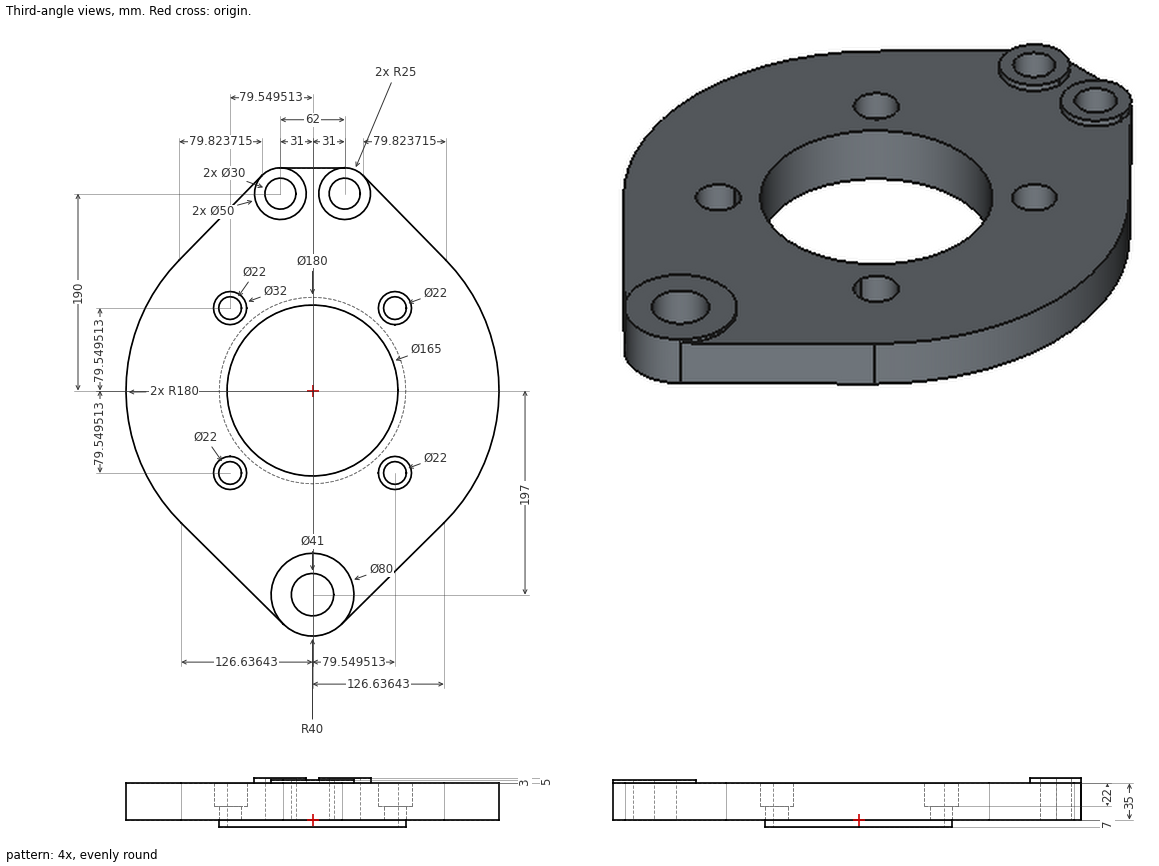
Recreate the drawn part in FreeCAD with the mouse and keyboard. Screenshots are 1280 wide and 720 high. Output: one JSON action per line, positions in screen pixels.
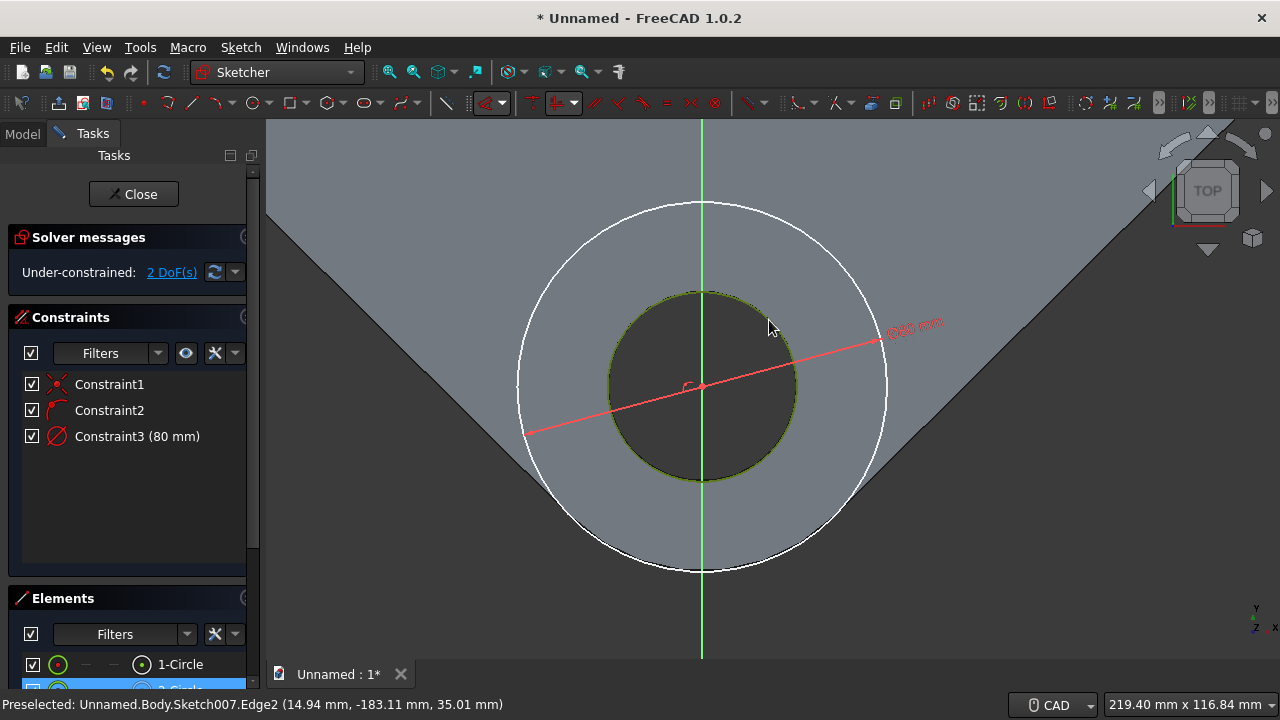
{"action": "key", "text": "k o"}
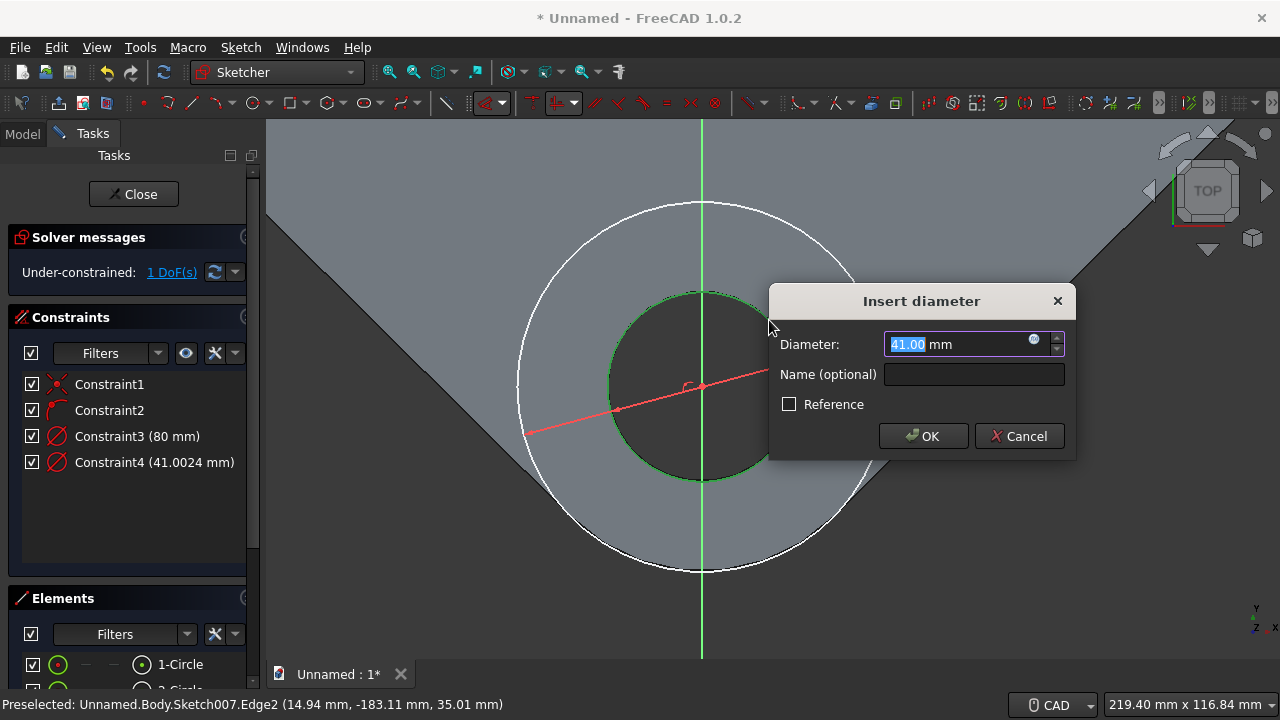
{"action": "type", "text": "41"}
{"action": "key", "text": "Return"}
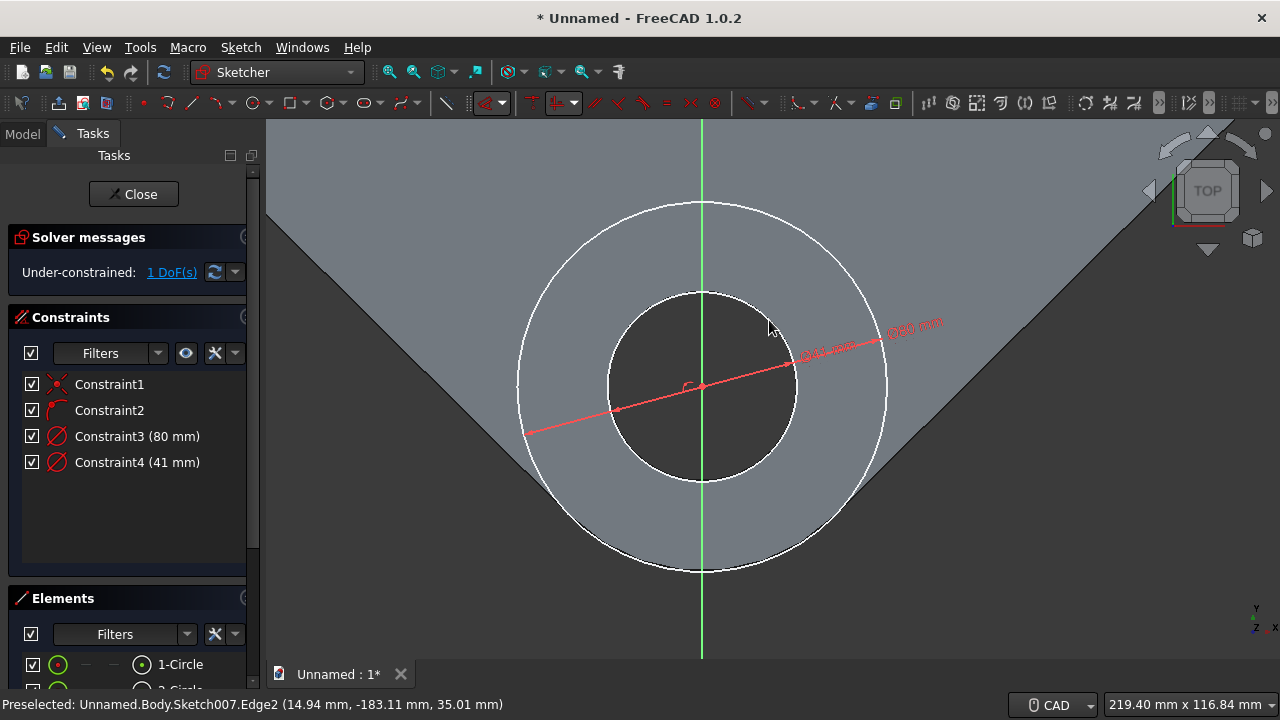
{"action": "left_click", "coordinate": [702, 387]}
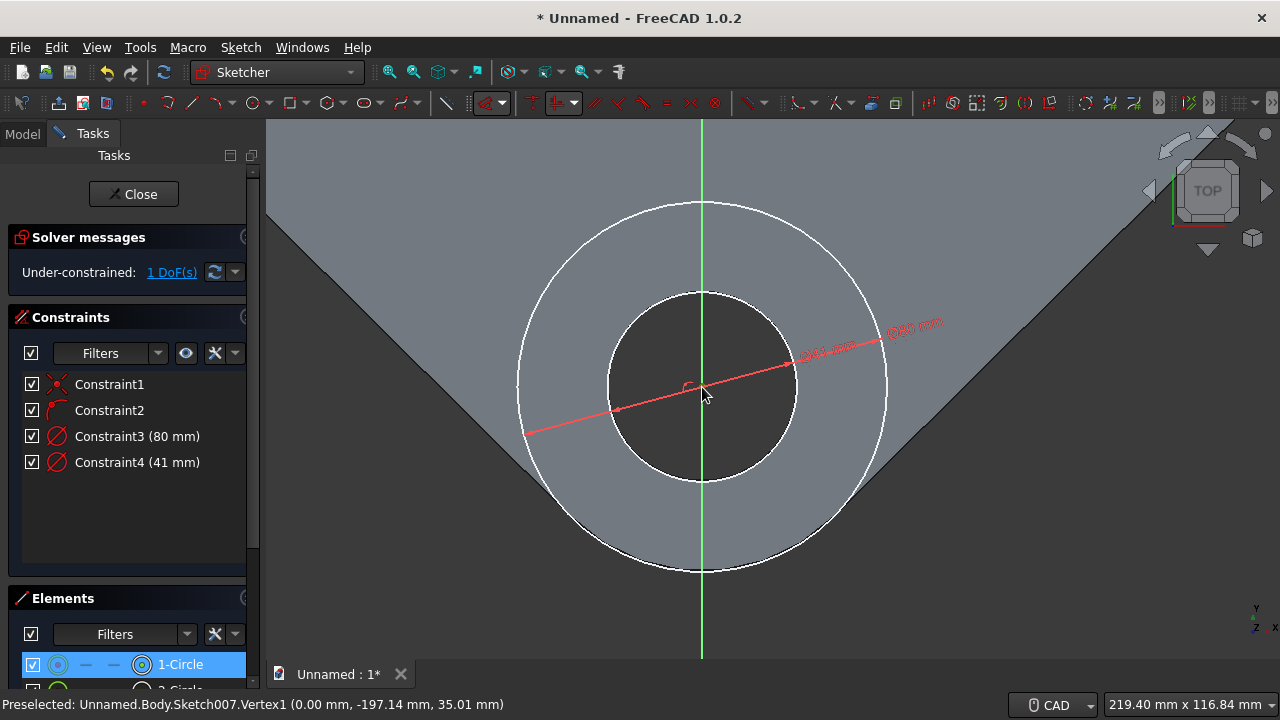
{"action": "key", "text": "i"}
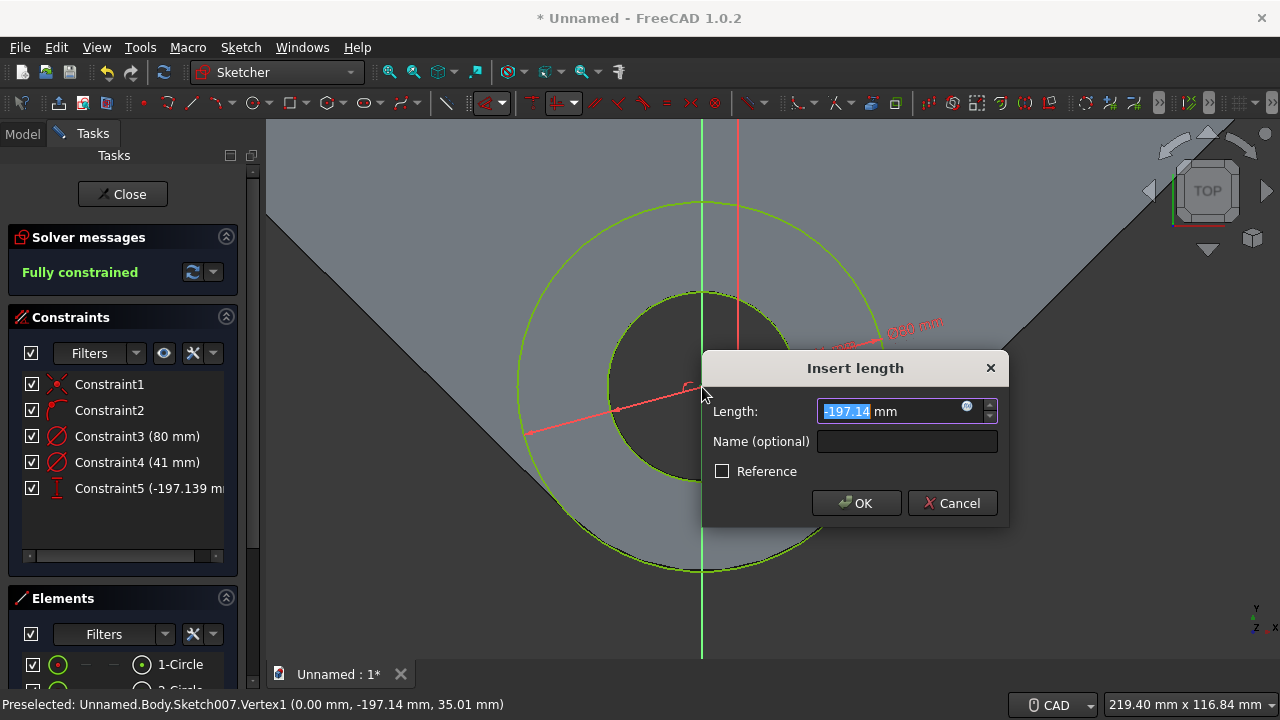
{"action": "type", "text": "-197"}
{"action": "key", "text": "Return"}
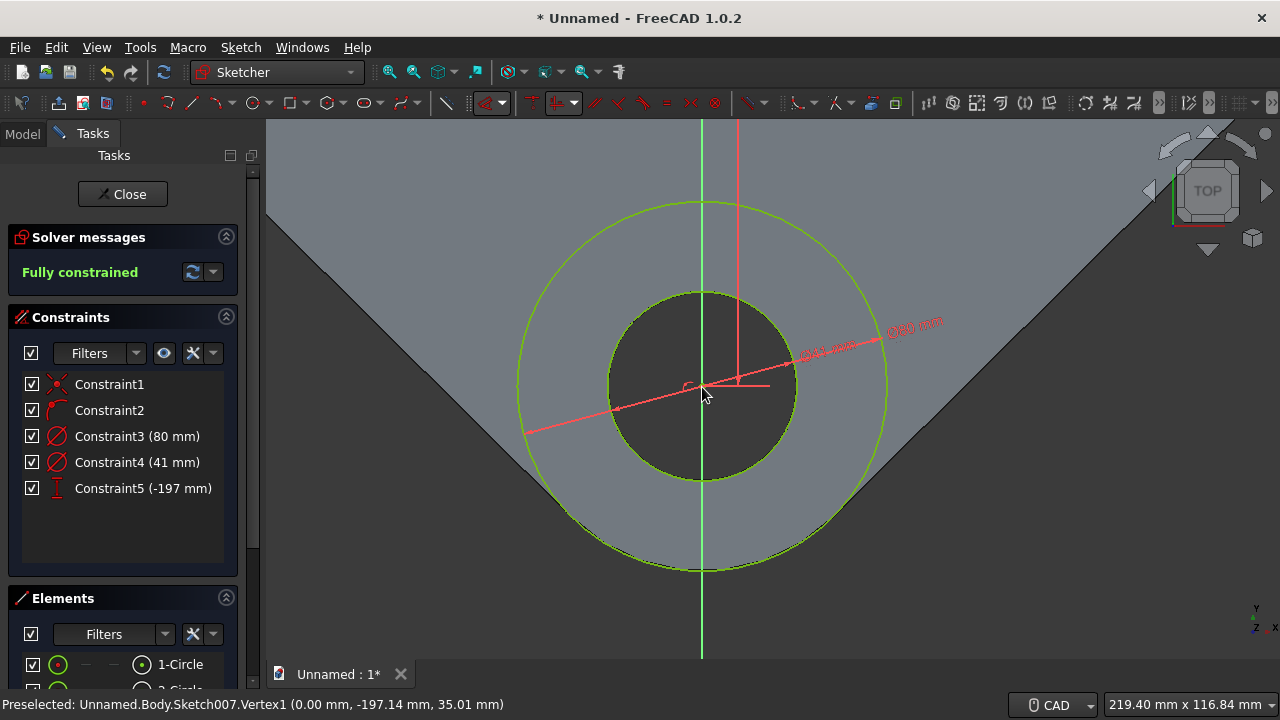
{"action": "left_click", "coordinate": [123, 194]}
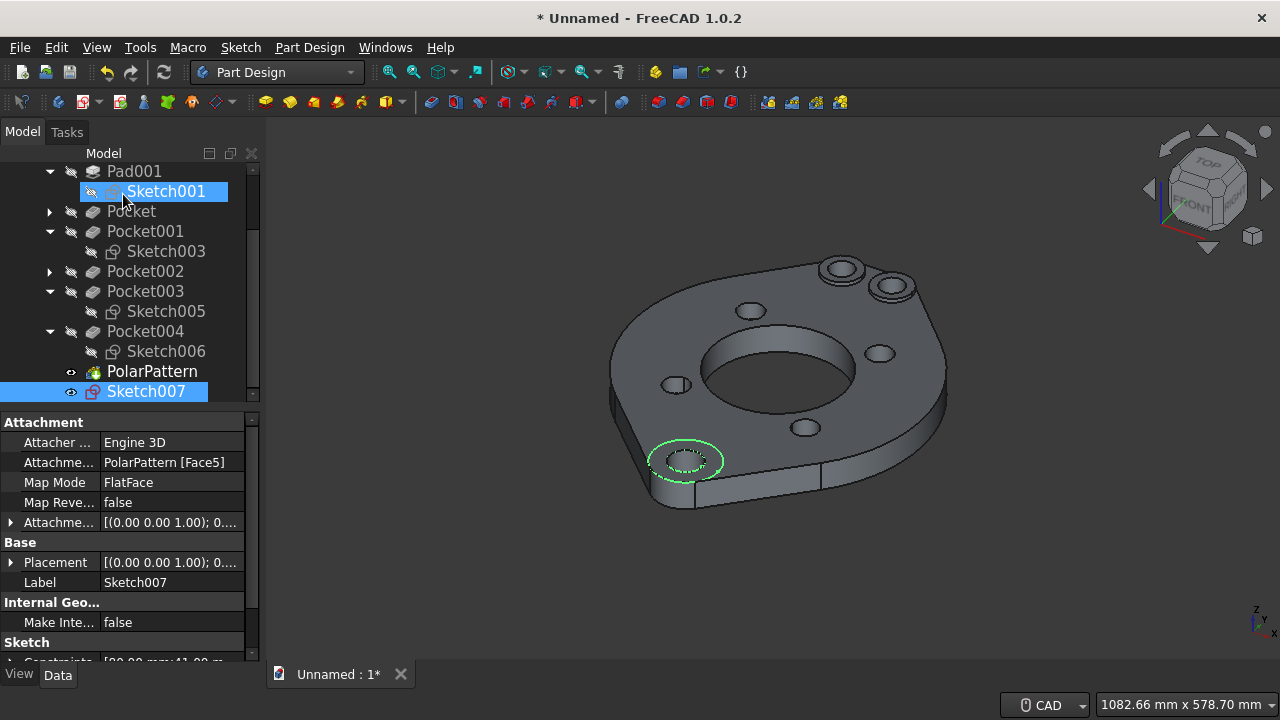
{"action": "left_click", "coordinate": [266, 102]}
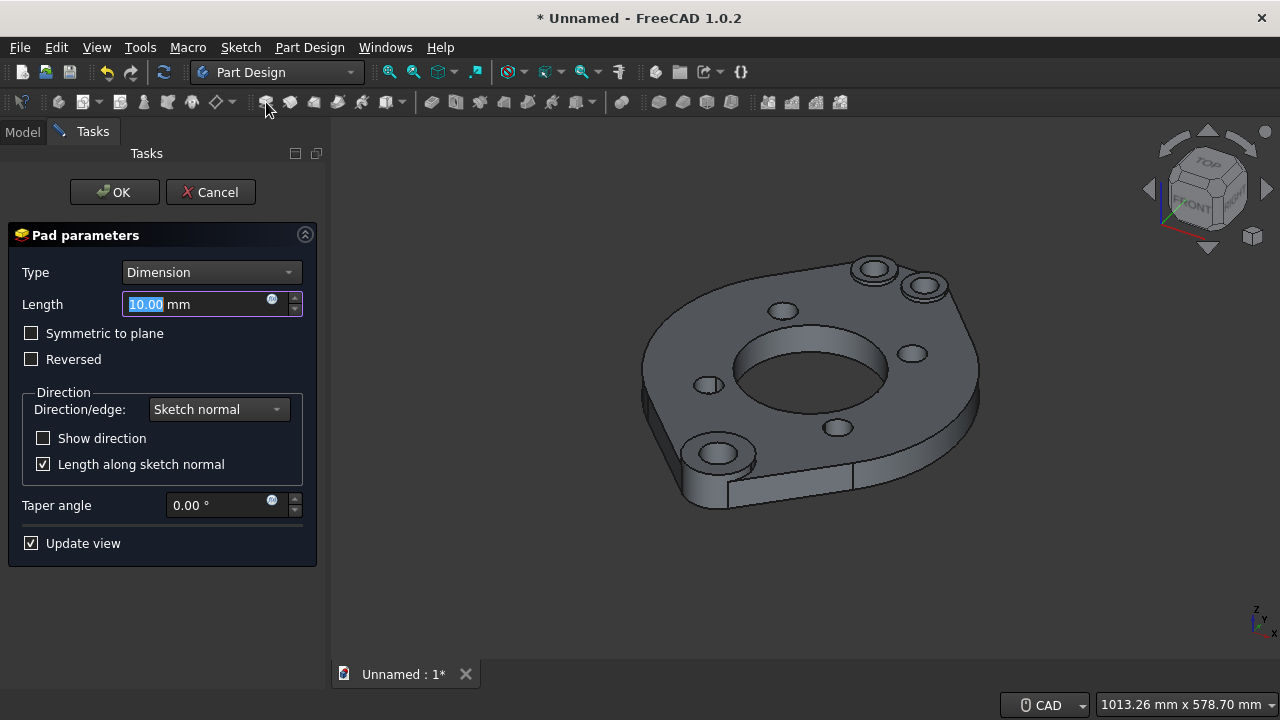
{"action": "type", "text": "3"}
{"action": "key", "text": "Tab"}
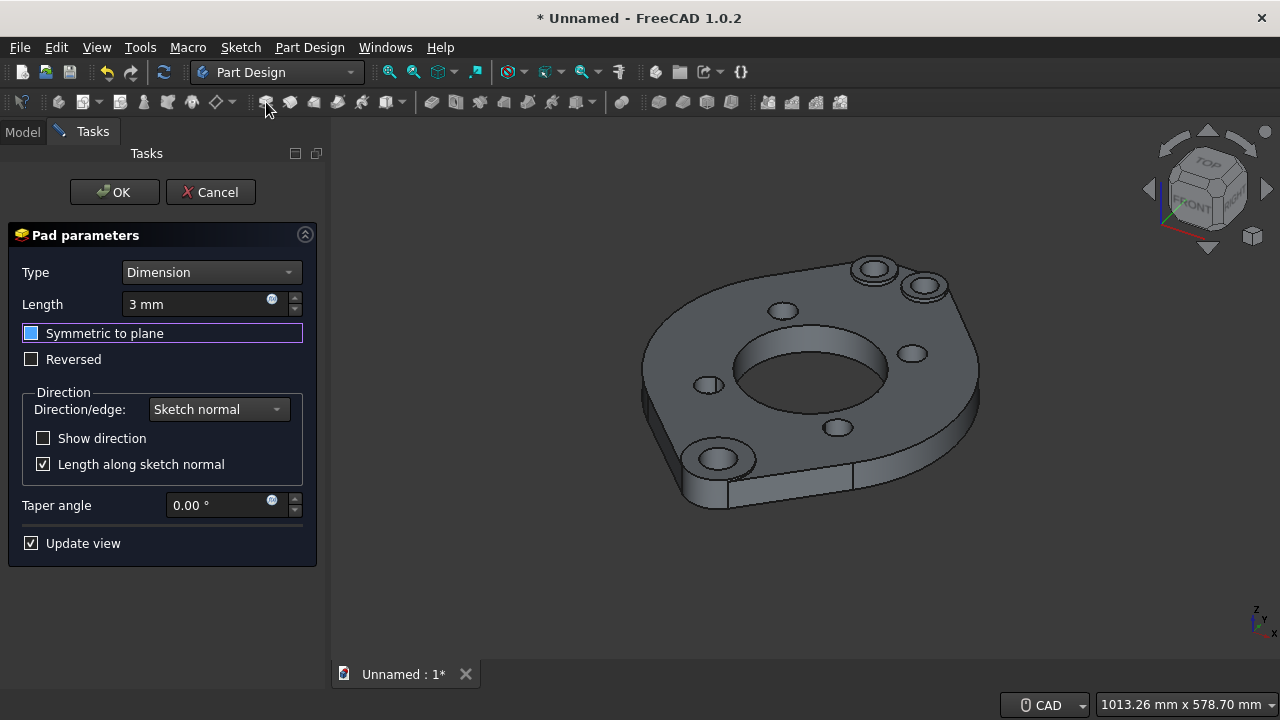
{"action": "left_click", "coordinate": [115, 192]}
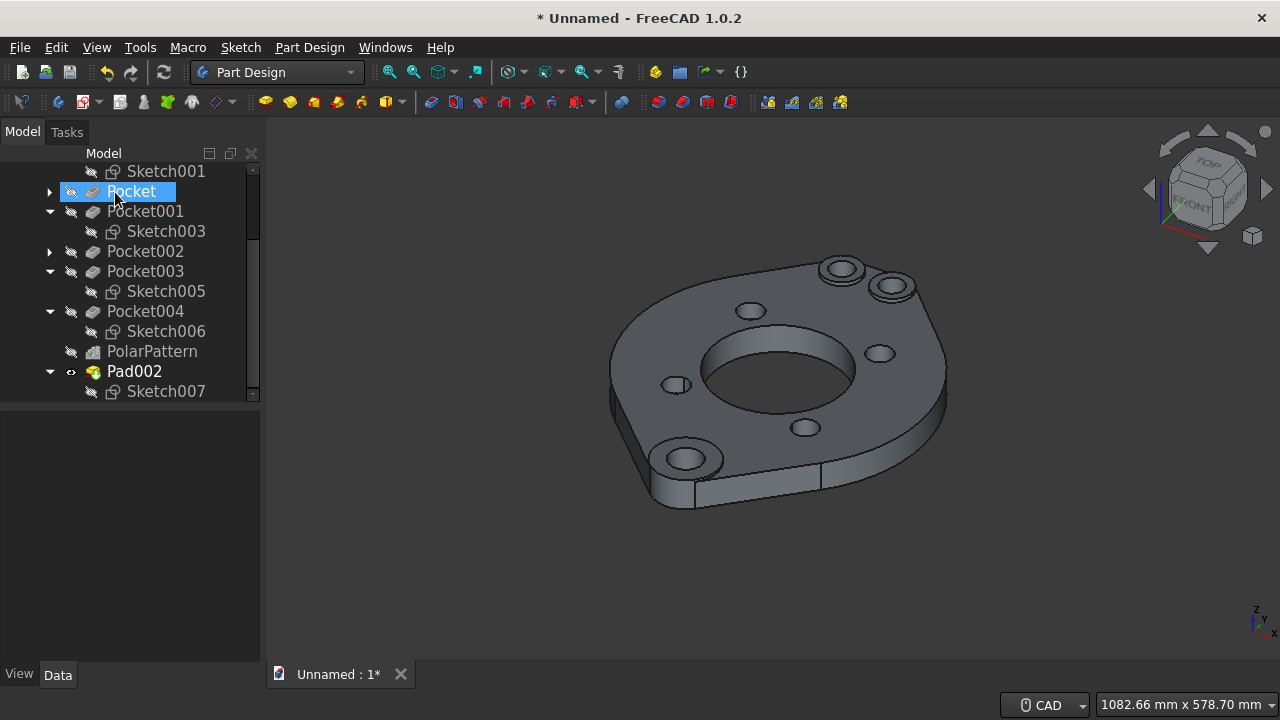
{"action": "scroll", "coordinate": [160, 287], "scroll_direction": "down", "scroll_amount": 3}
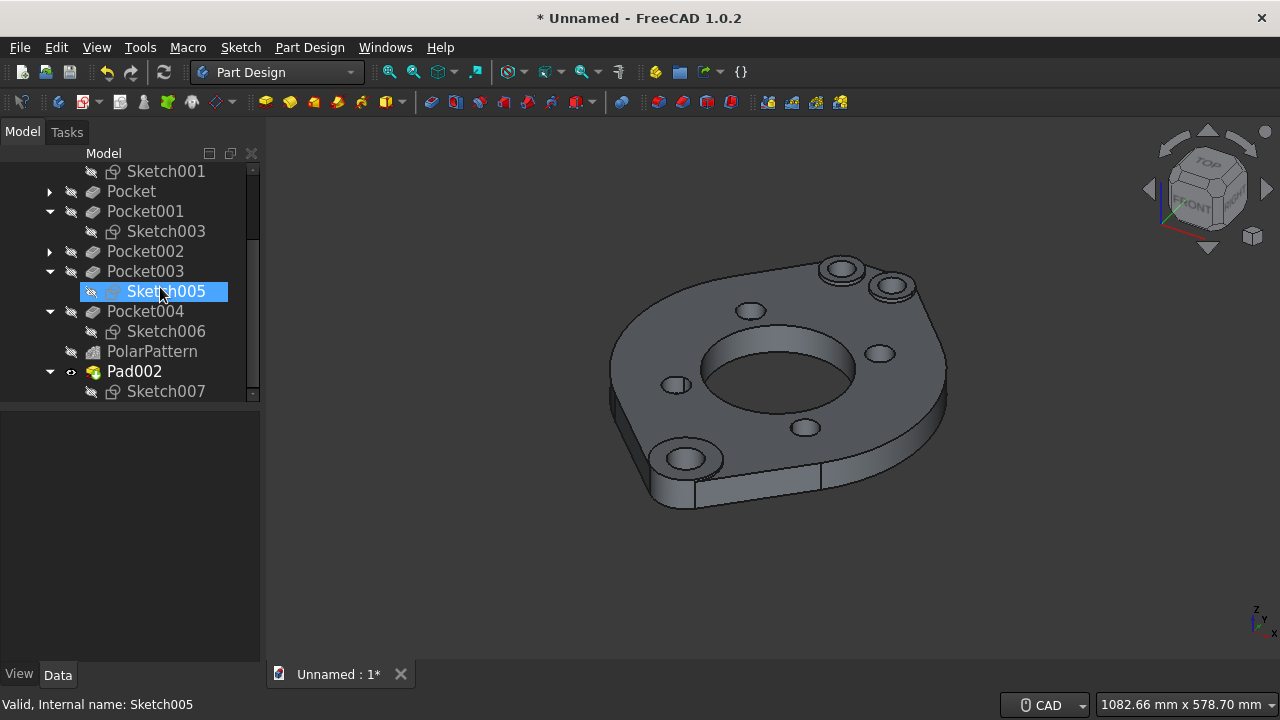
{"action": "scroll", "coordinate": [160, 287], "scroll_direction": "up", "scroll_amount": 15}